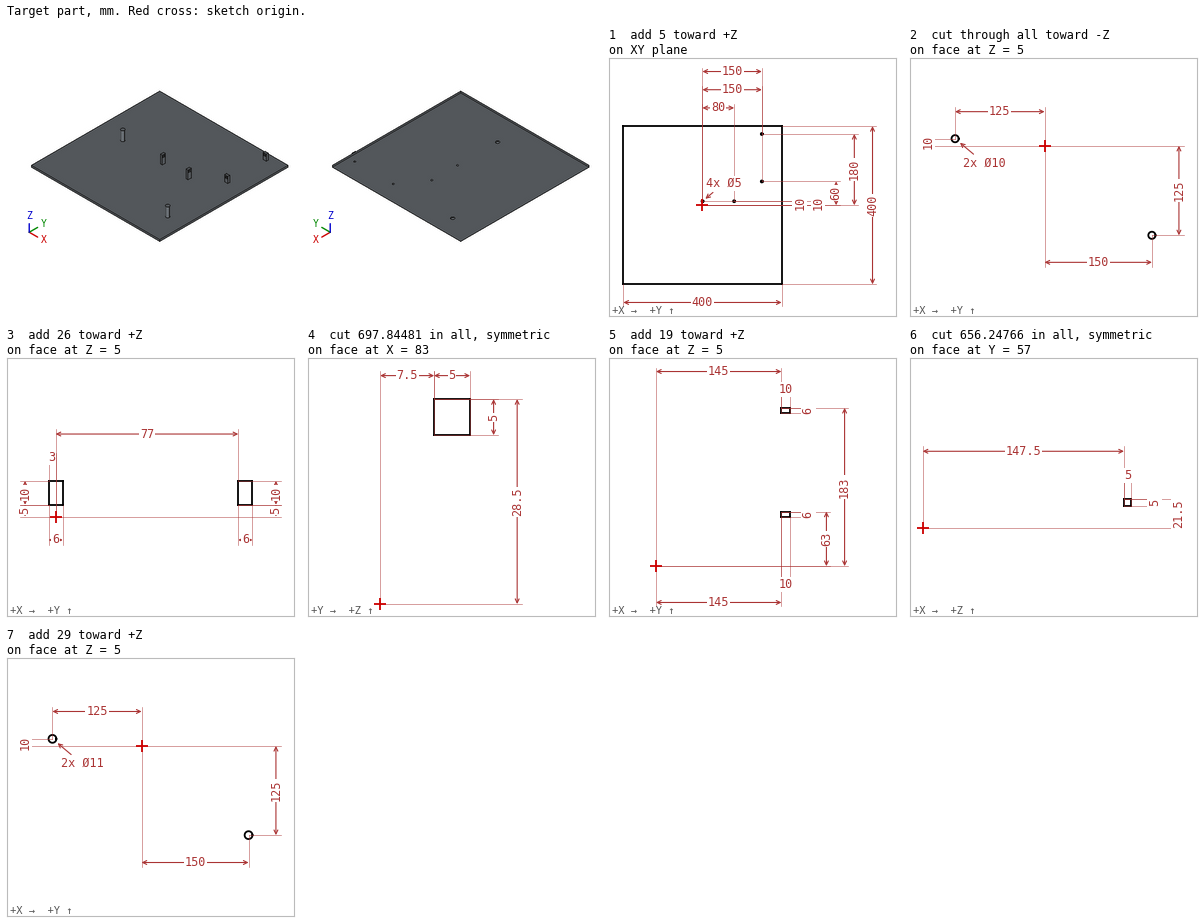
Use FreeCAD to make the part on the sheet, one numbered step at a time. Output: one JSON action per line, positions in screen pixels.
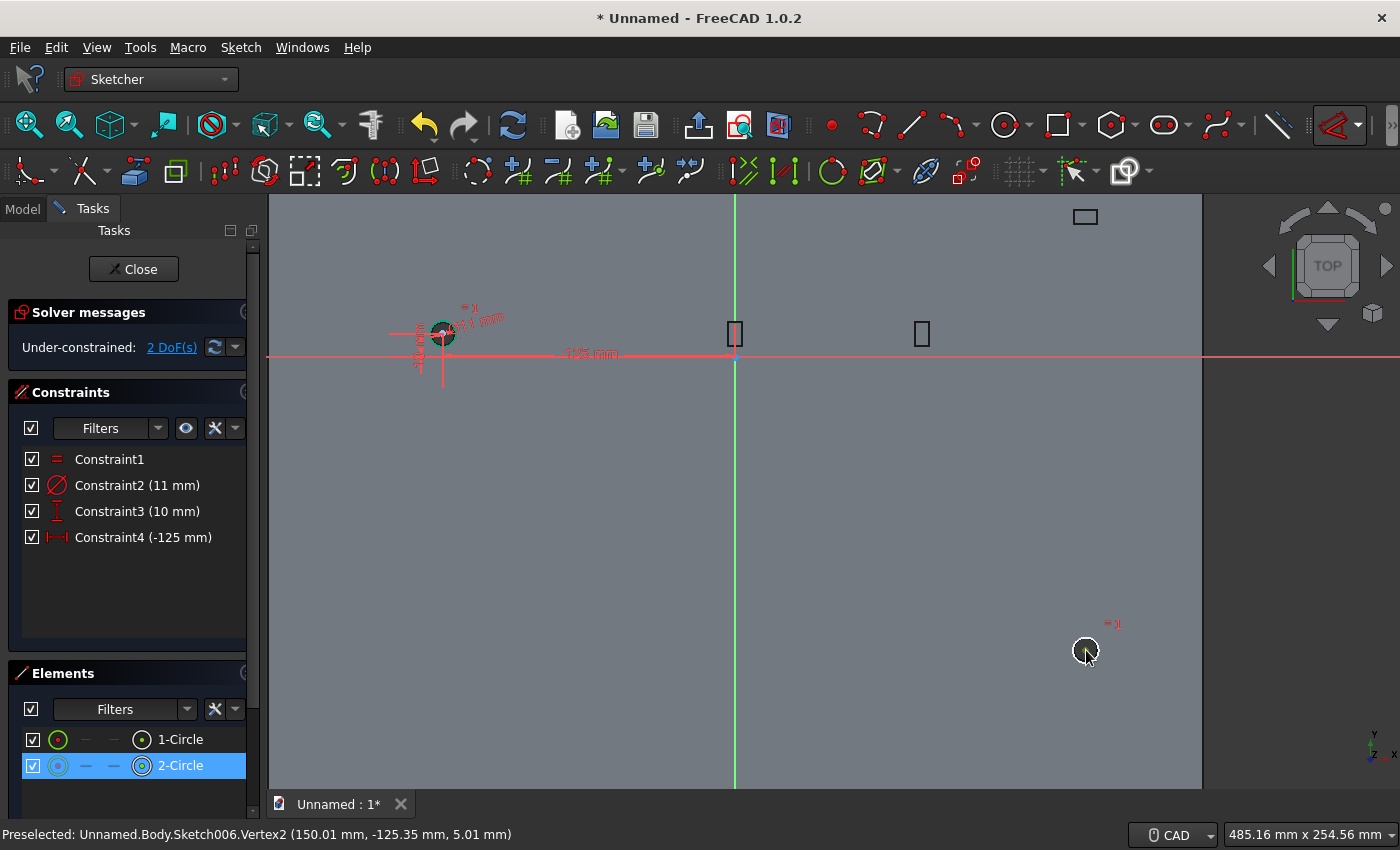
{"action": "key", "text": "l"}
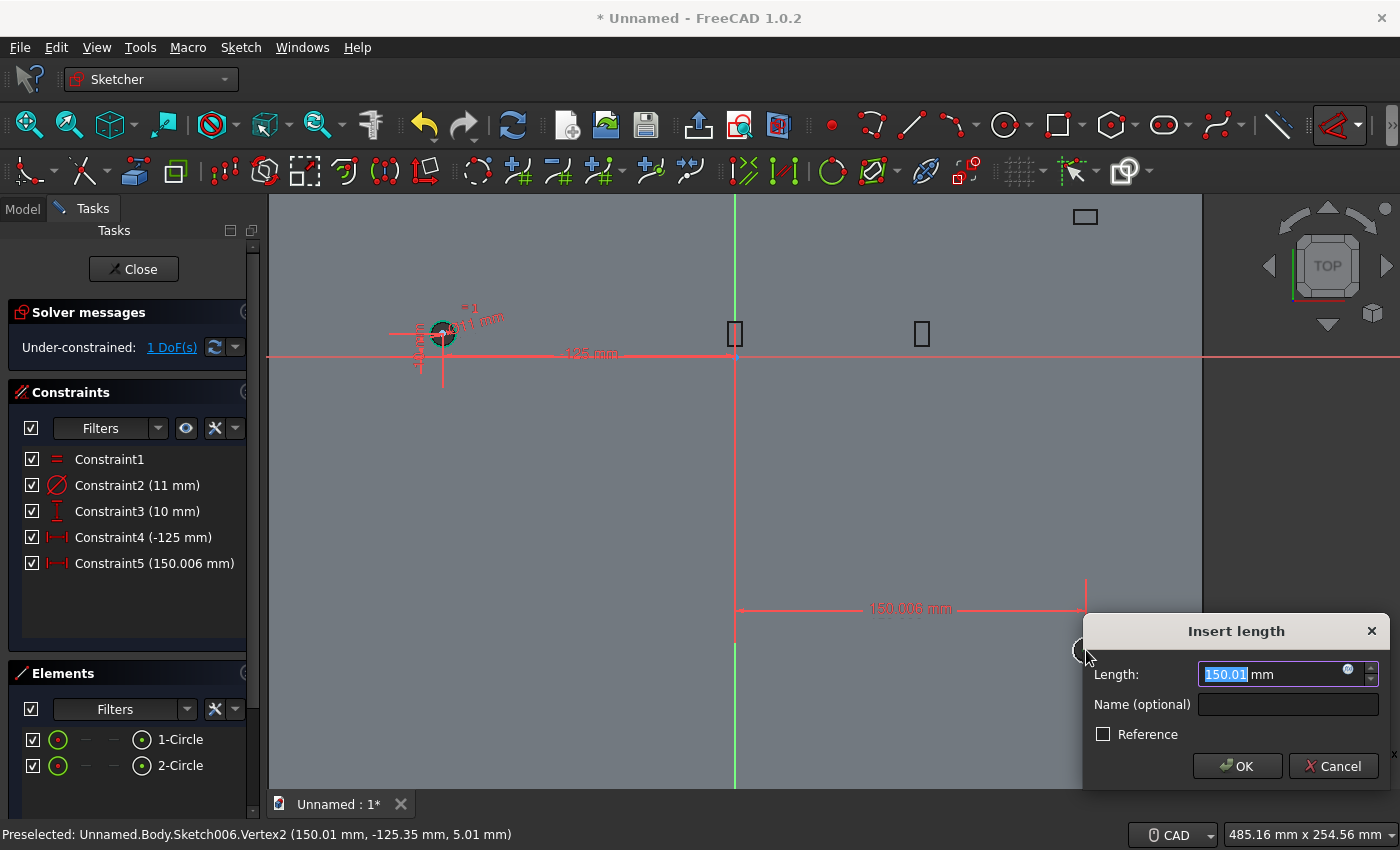
{"action": "type", "text": "150"}
{"action": "key", "text": "Return"}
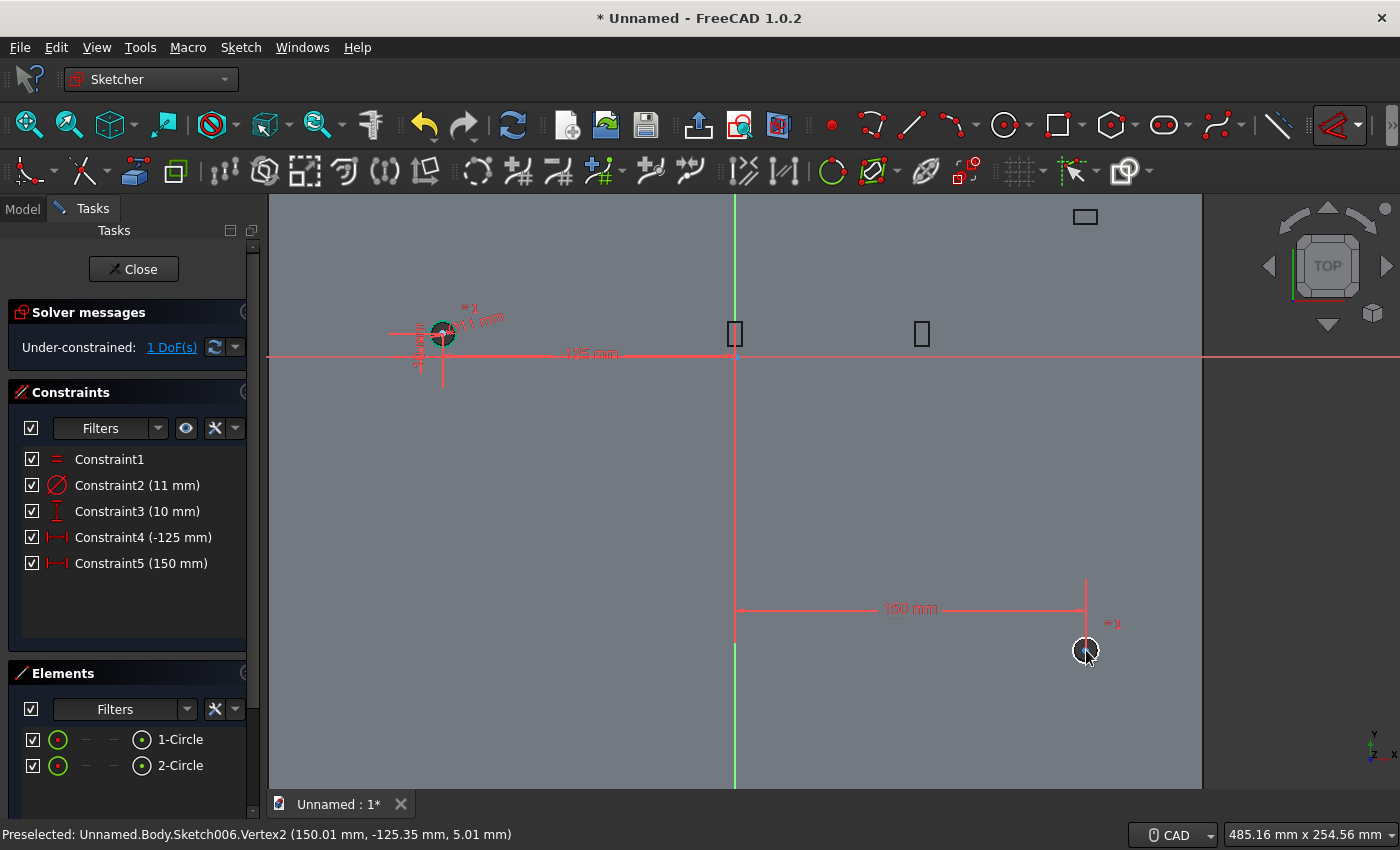
{"action": "left_click", "coordinate": [1086, 650]}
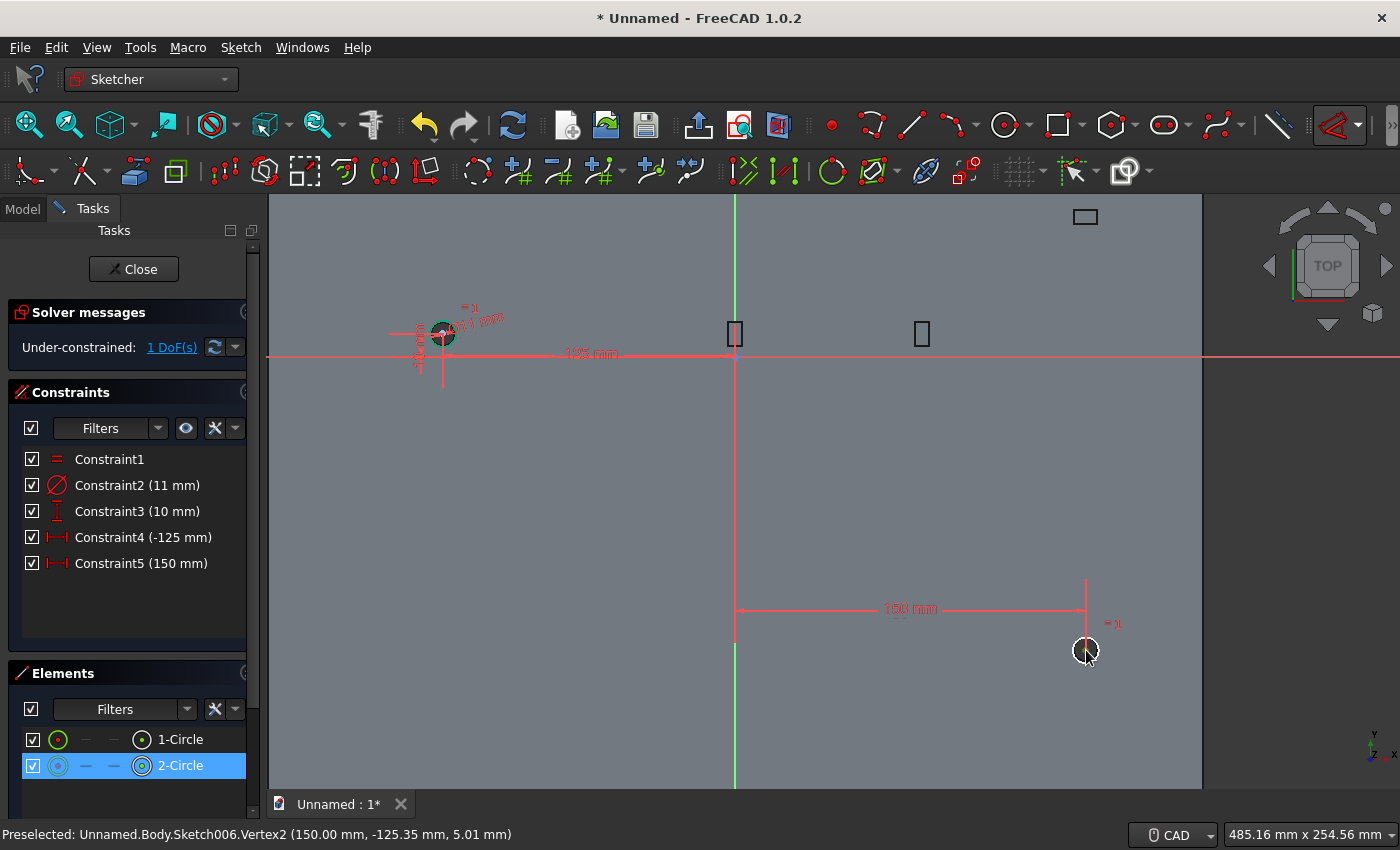
{"action": "key", "text": "i"}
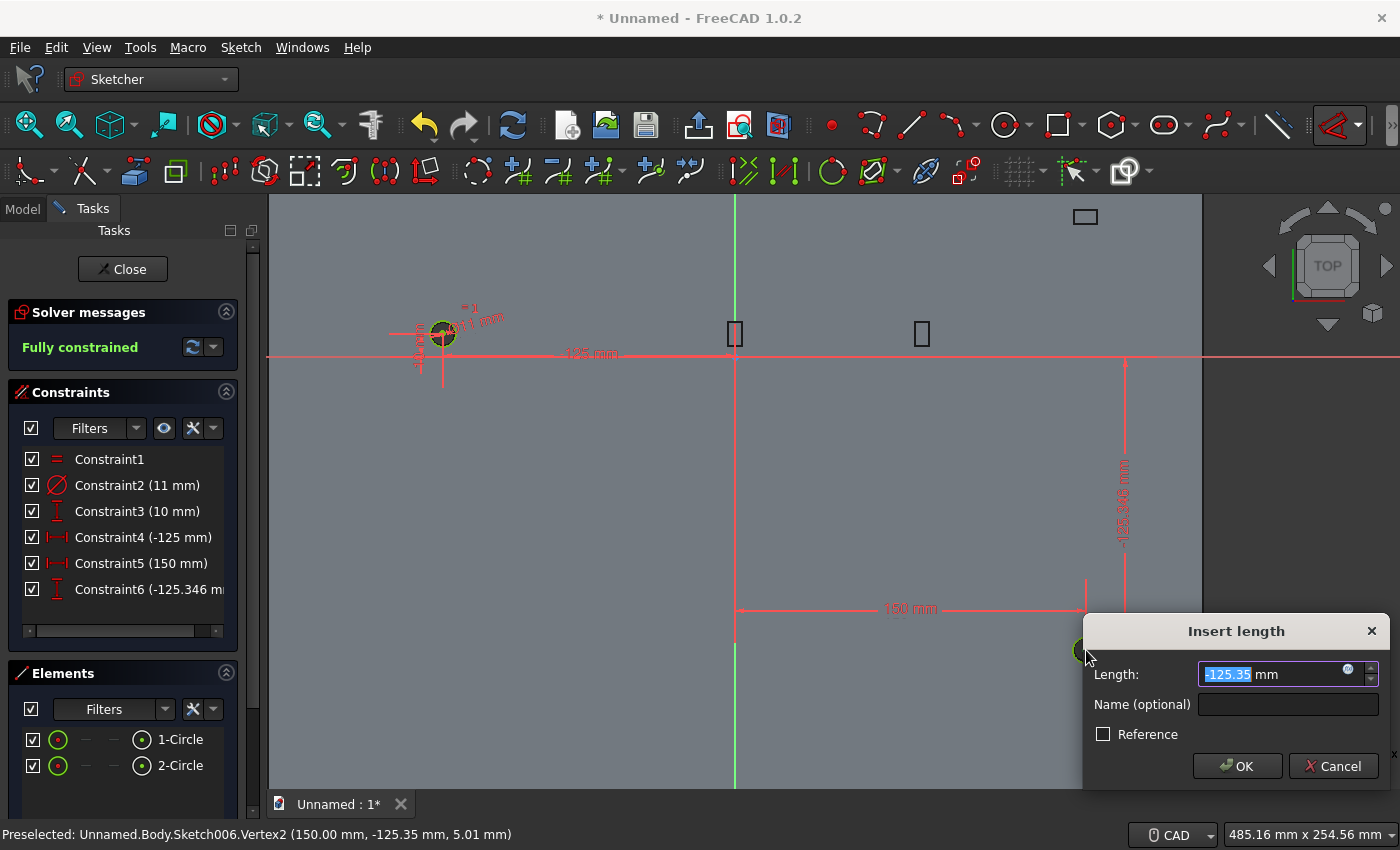
{"action": "type", "text": "-125"}
{"action": "key", "text": "Return"}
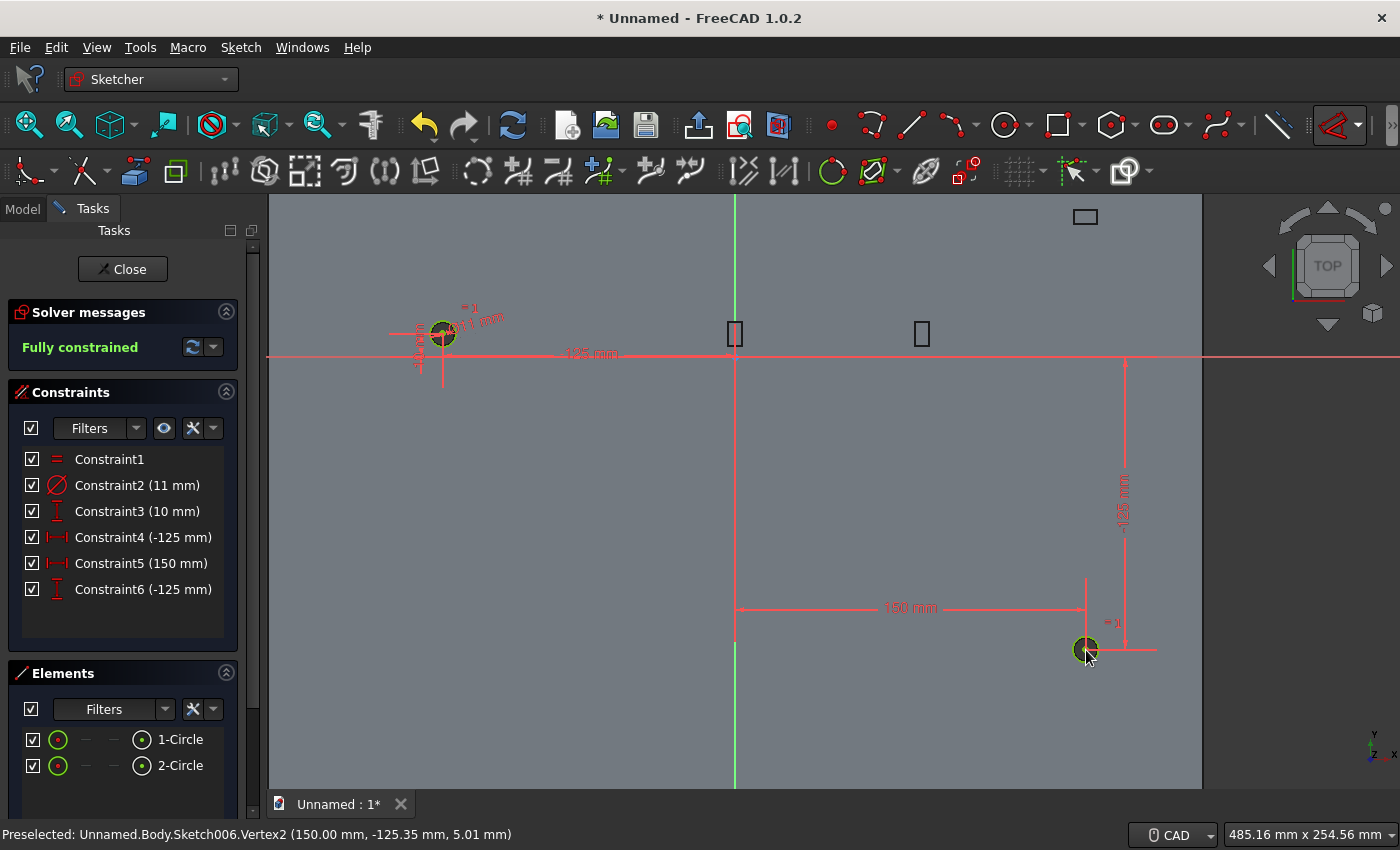
{"action": "left_click", "coordinate": [123, 269]}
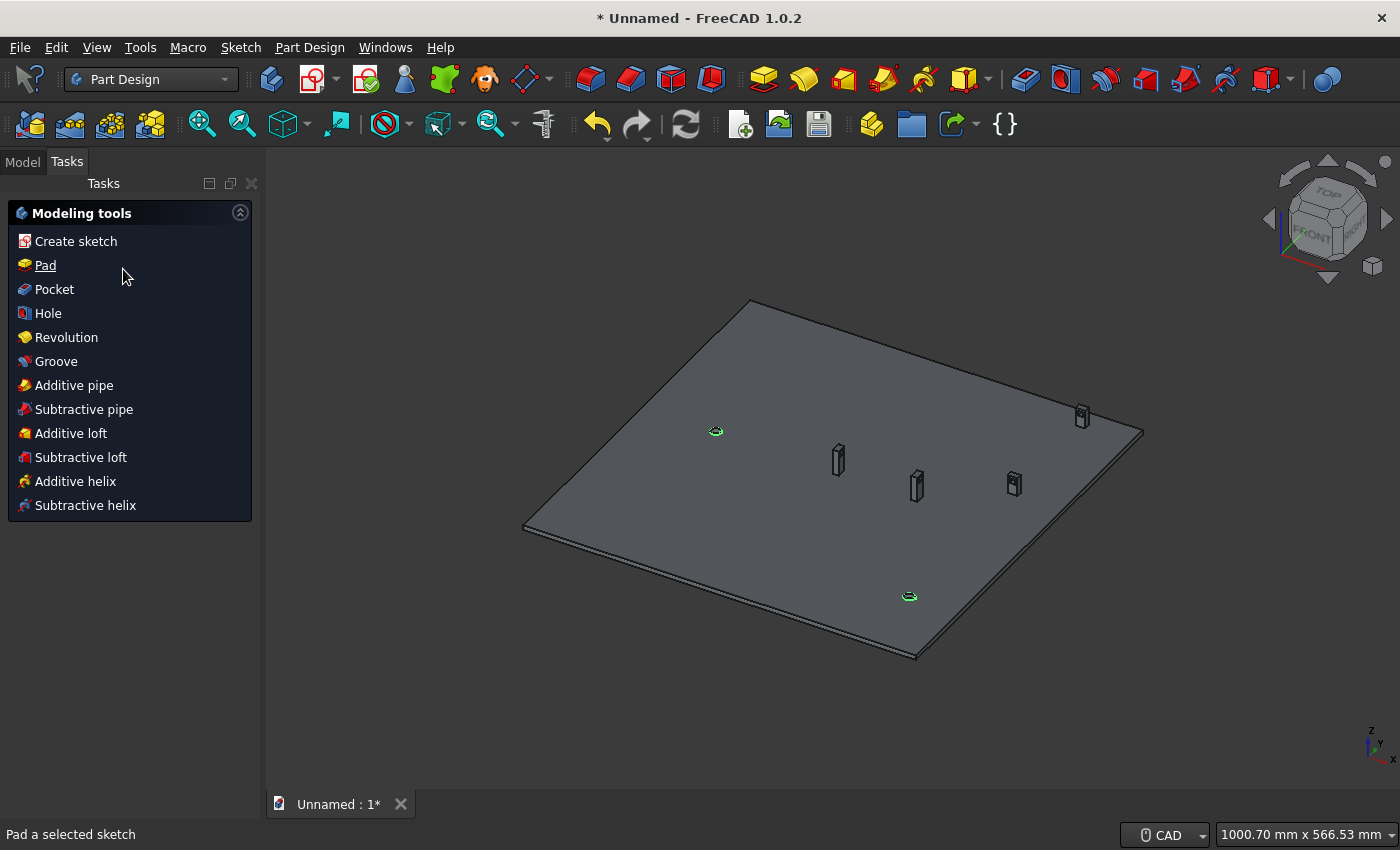
{"action": "left_click", "coordinate": [764, 80]}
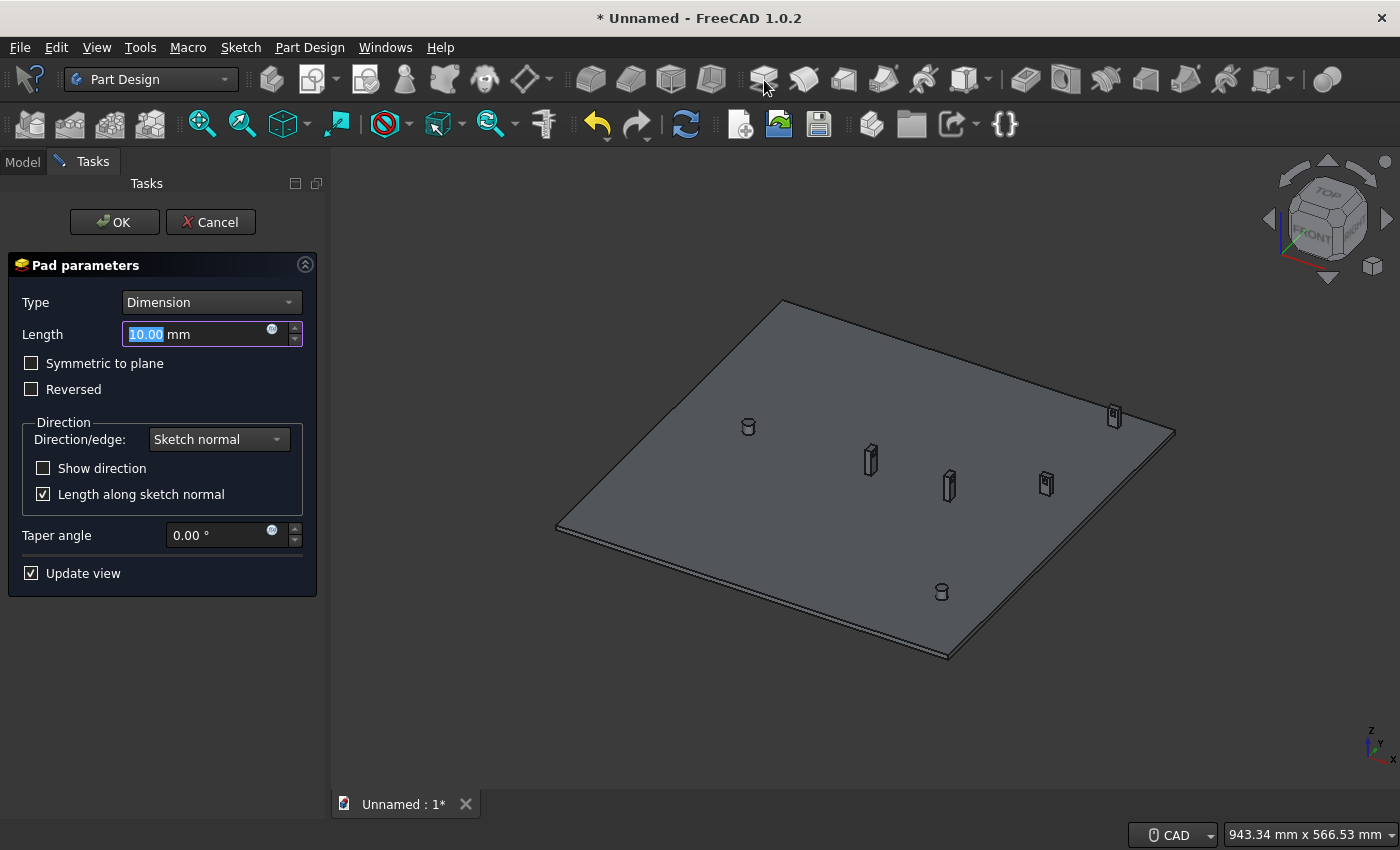
{"action": "type", "text": "29"}
{"action": "key", "text": "Tab"}